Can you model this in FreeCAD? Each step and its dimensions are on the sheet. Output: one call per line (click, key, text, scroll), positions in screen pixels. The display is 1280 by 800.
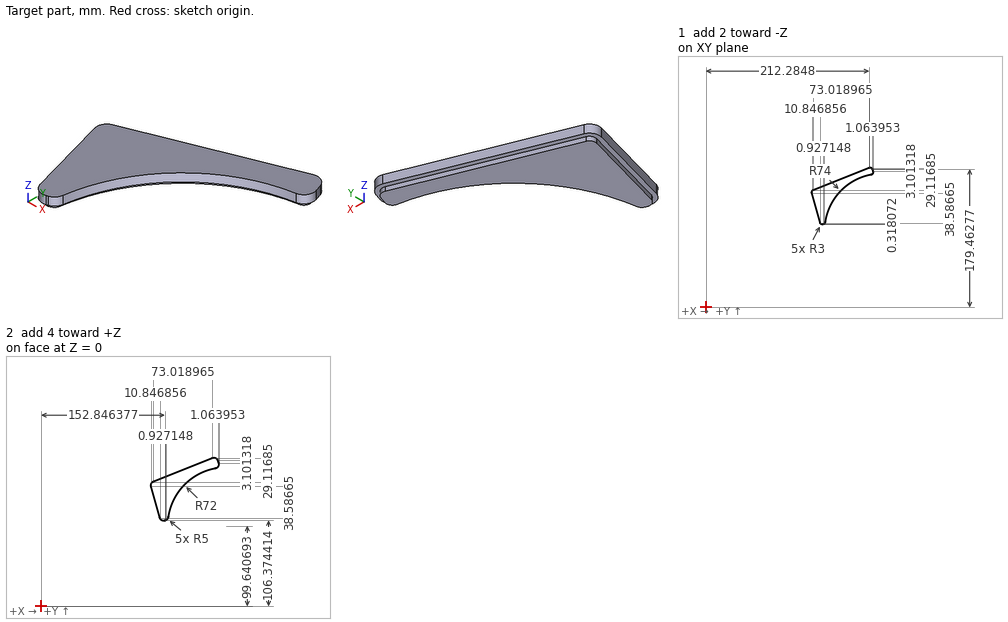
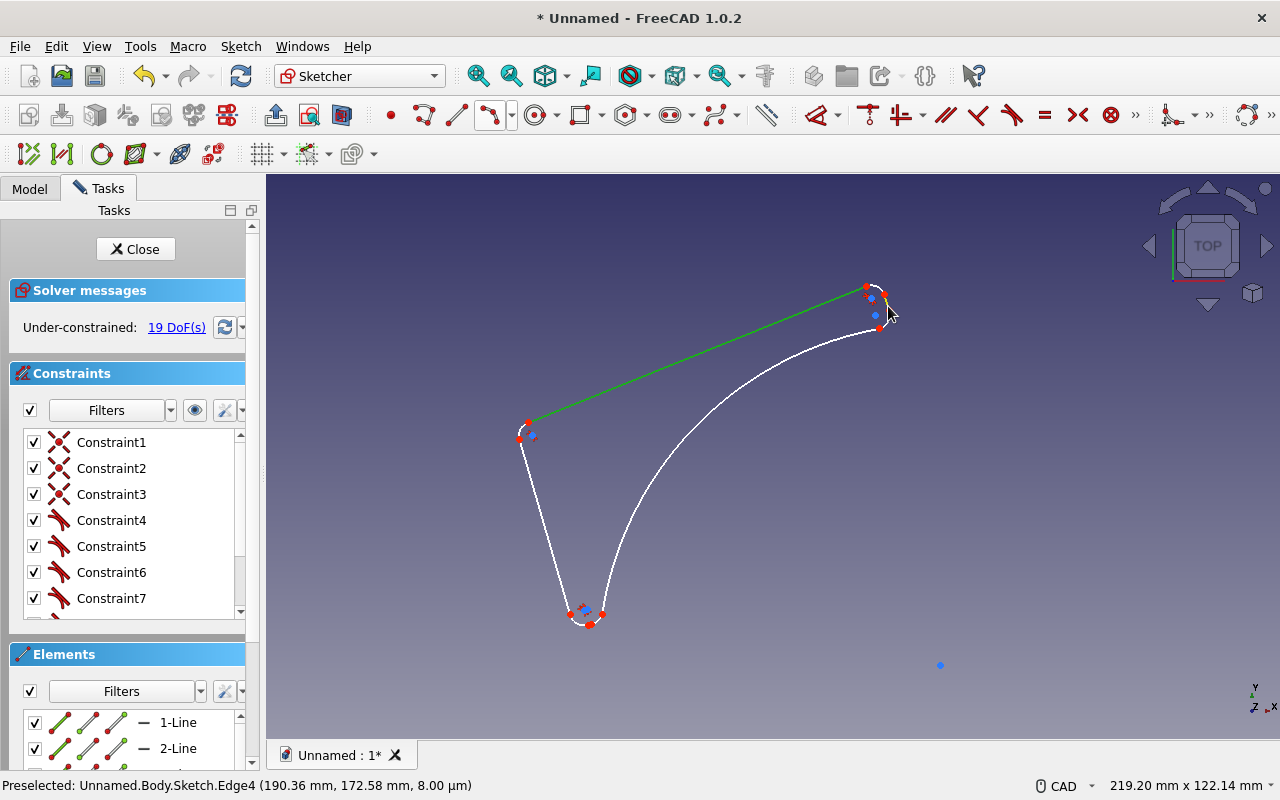
scroll(523, 426, up, 5)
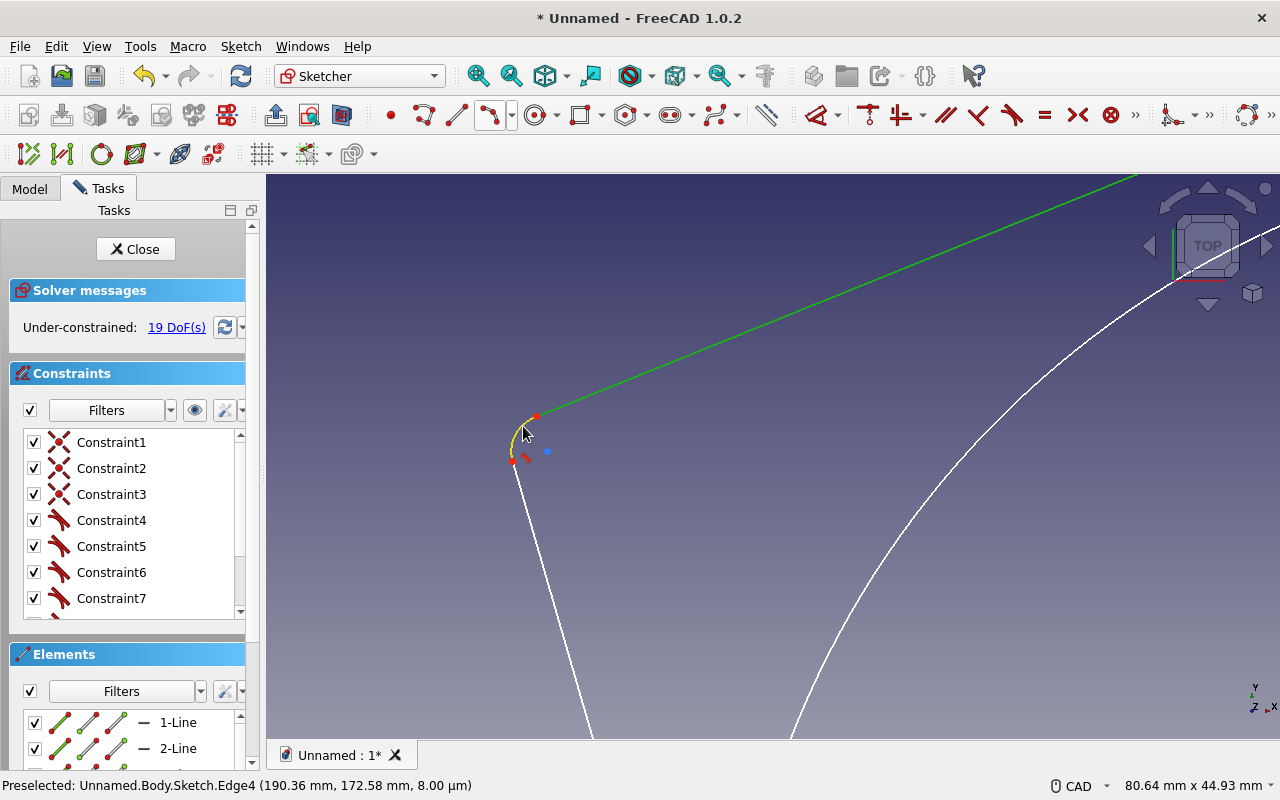
click(522, 425)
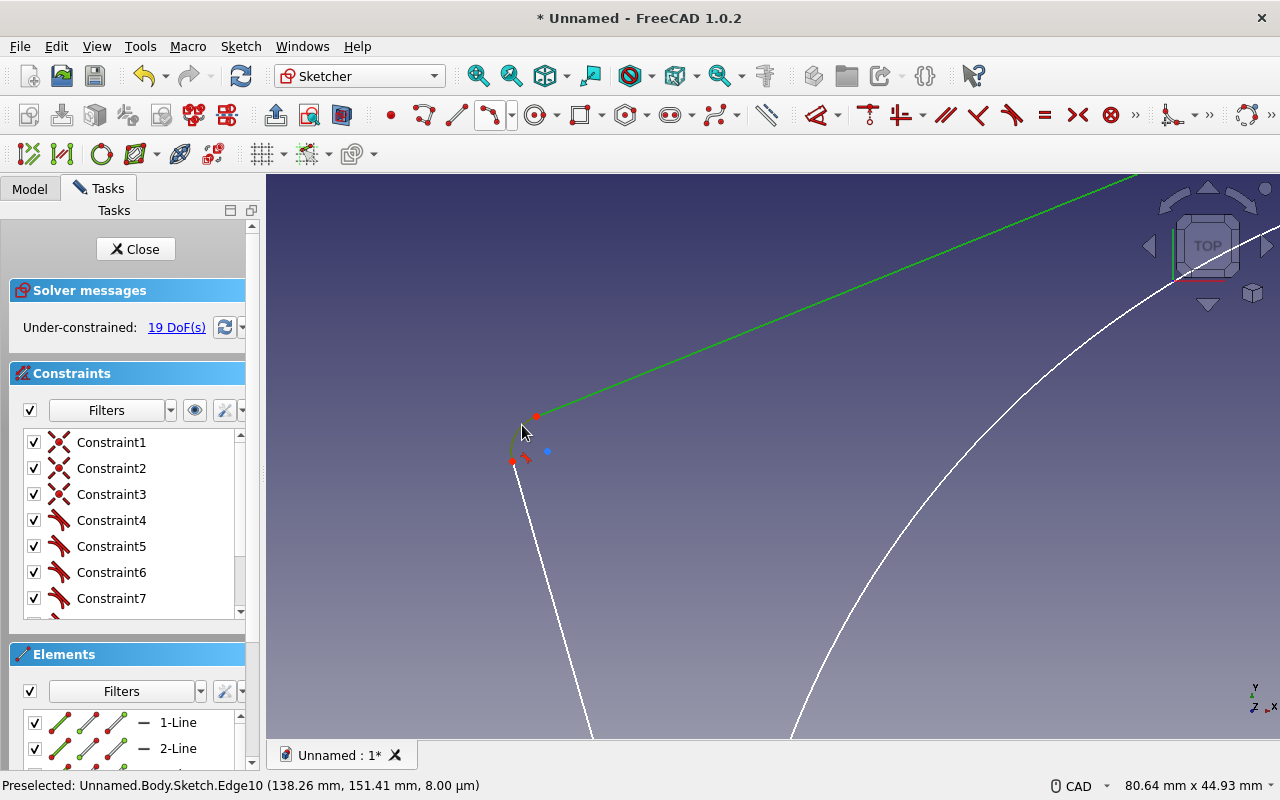
click(1012, 116)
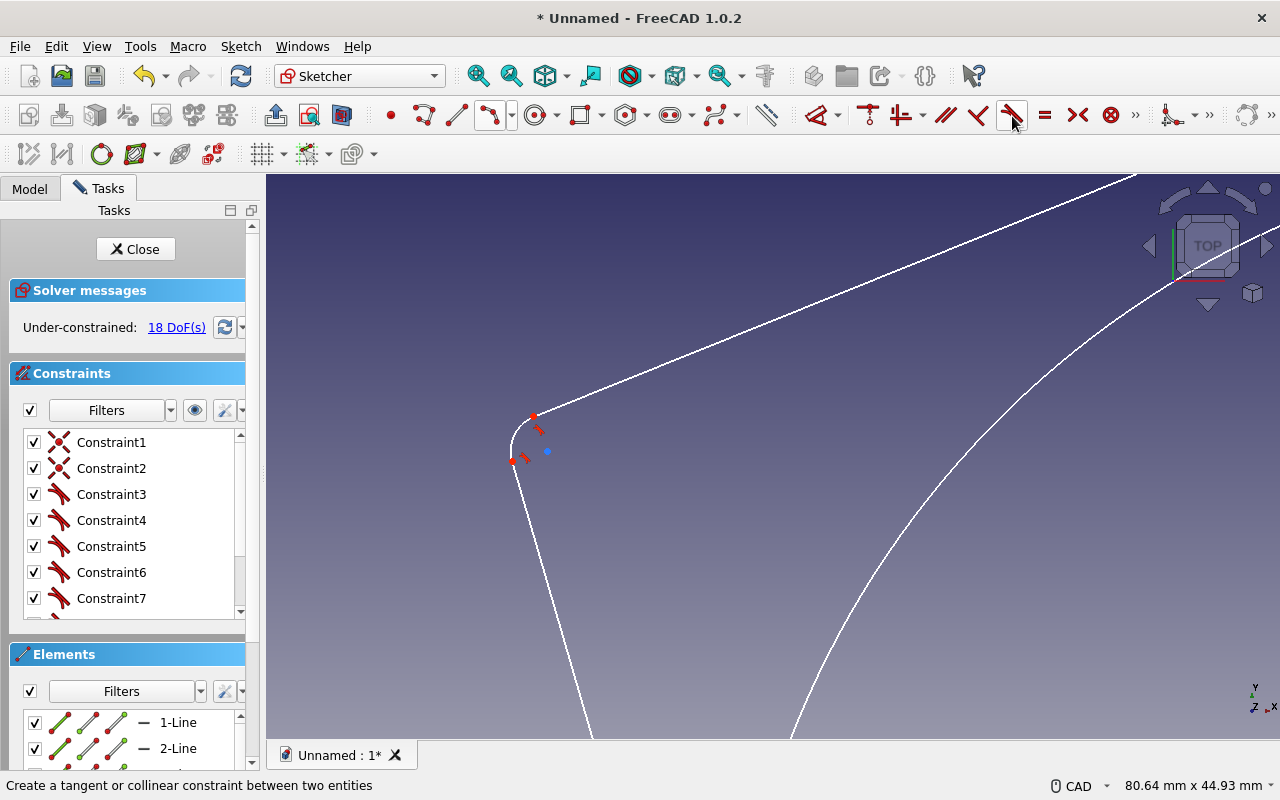
scroll(523, 426, down, 5)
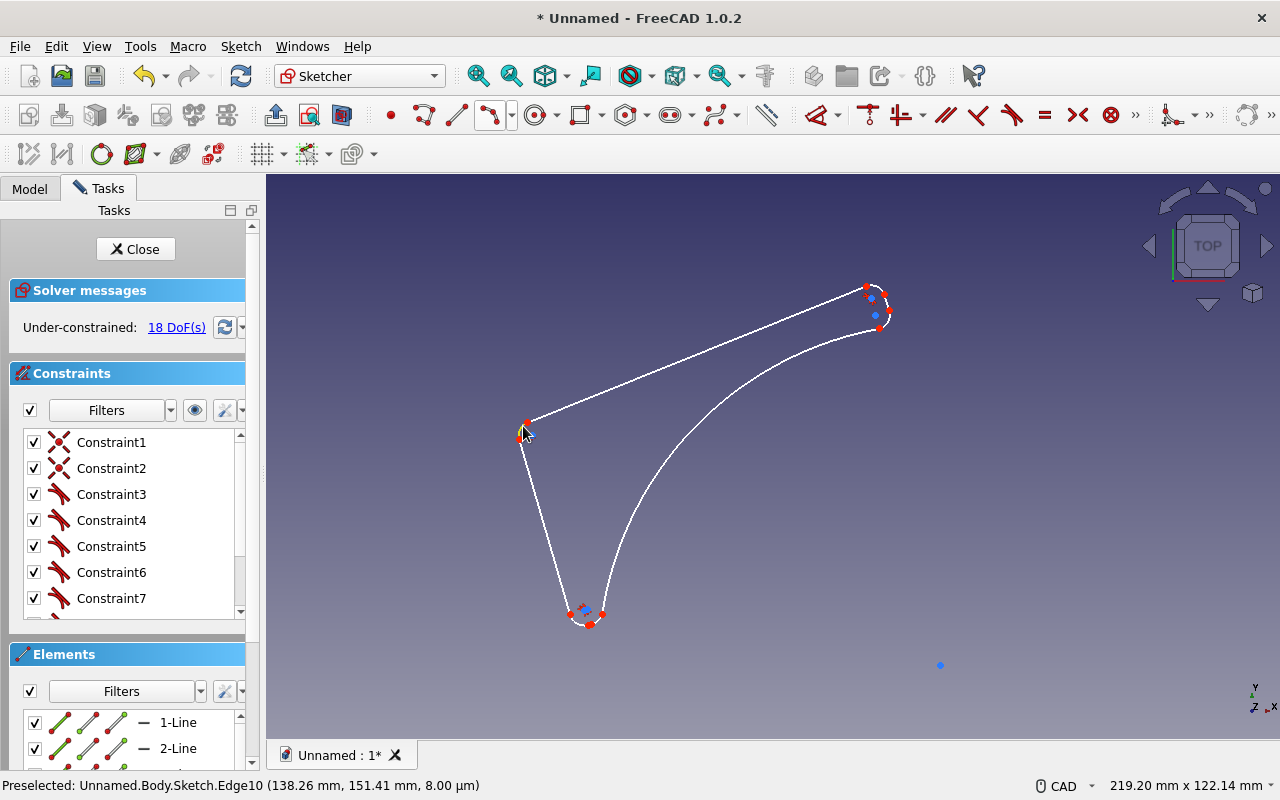
scroll(596, 622, up, 6)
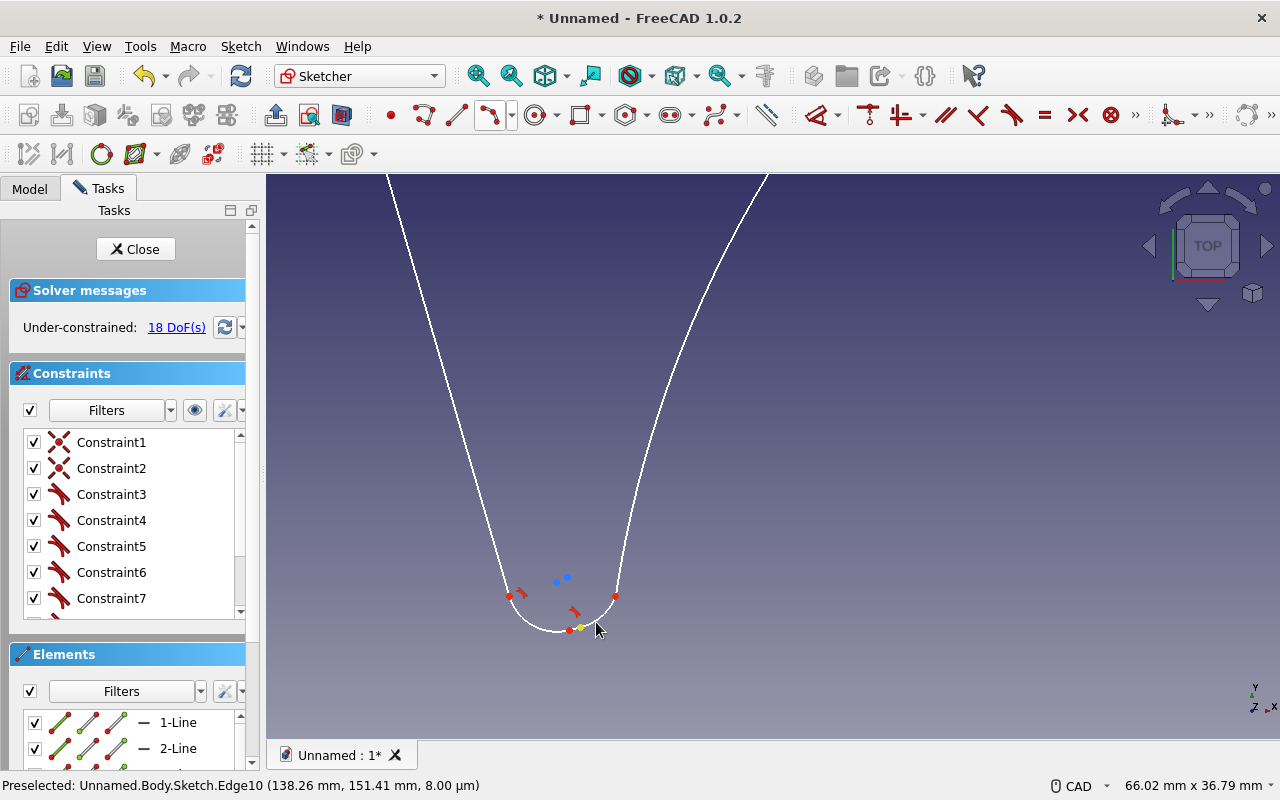
click(594, 622)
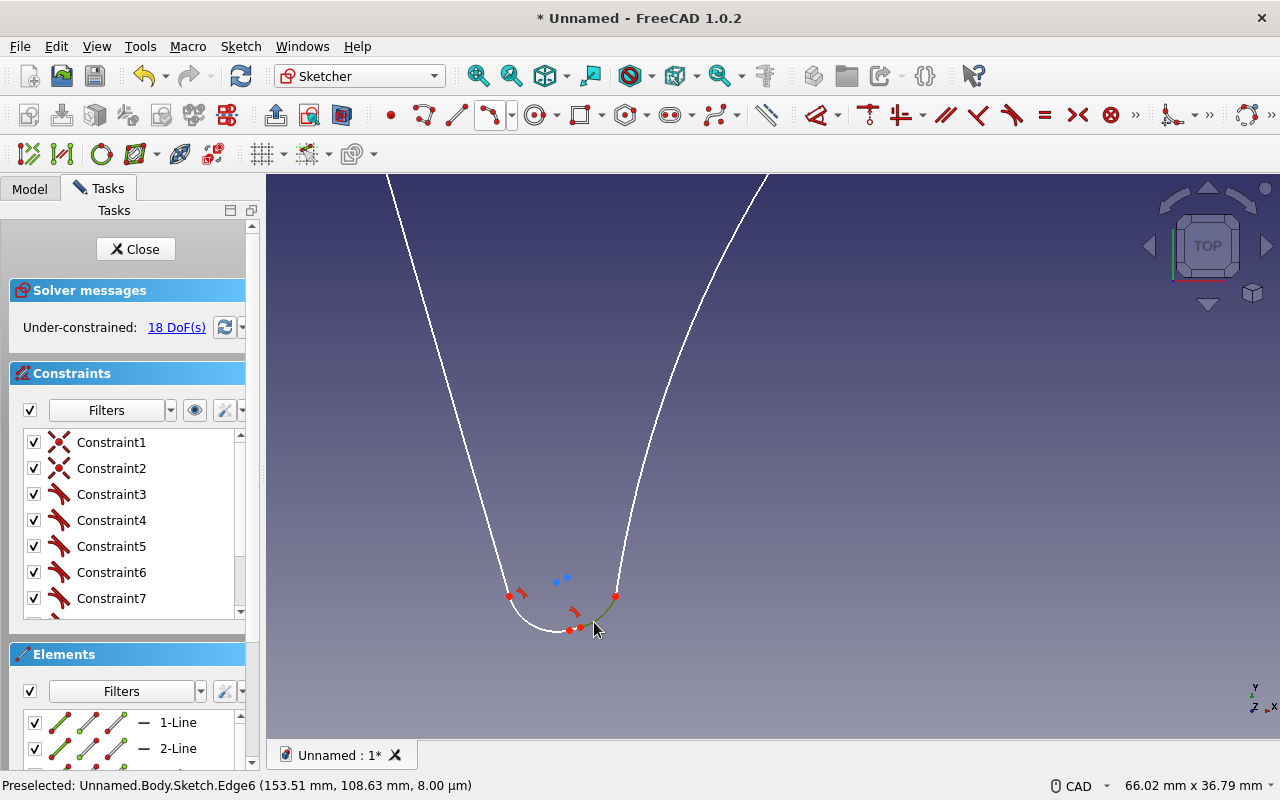
click(691, 325)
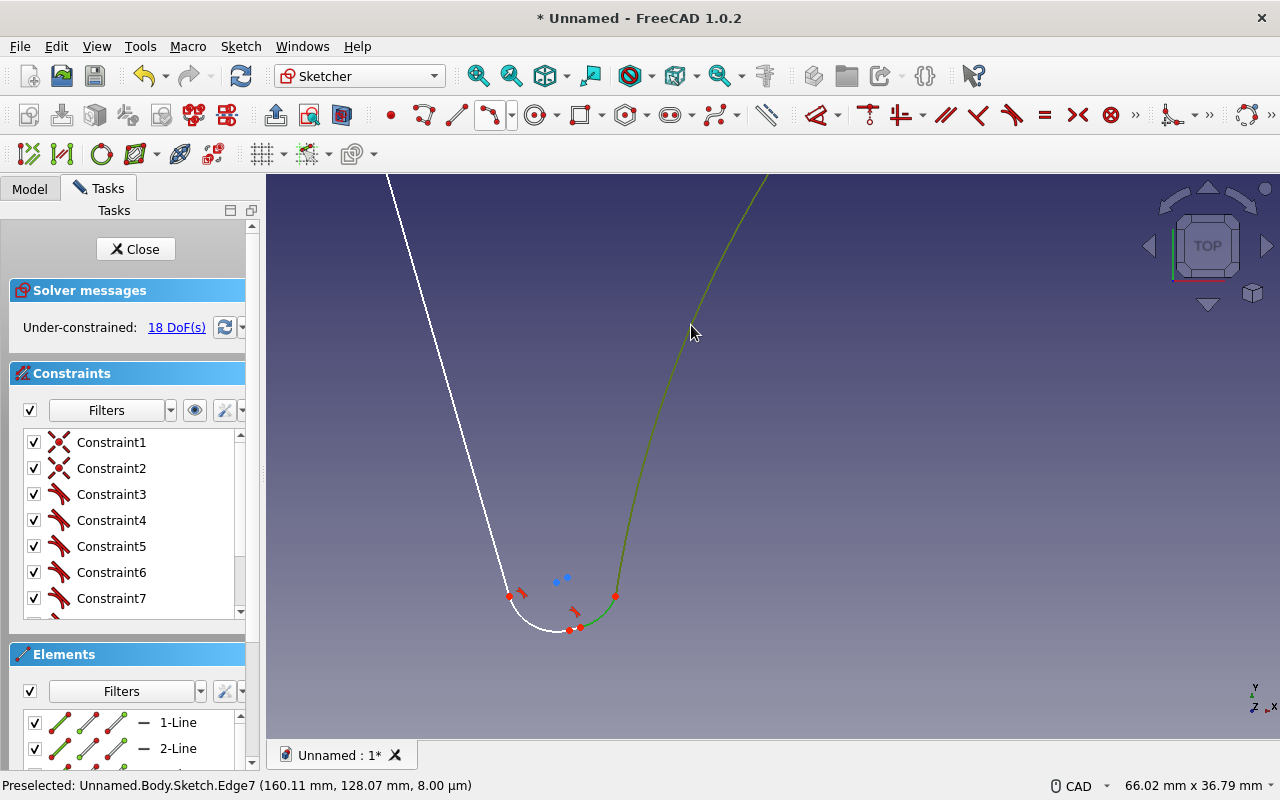
click(1012, 116)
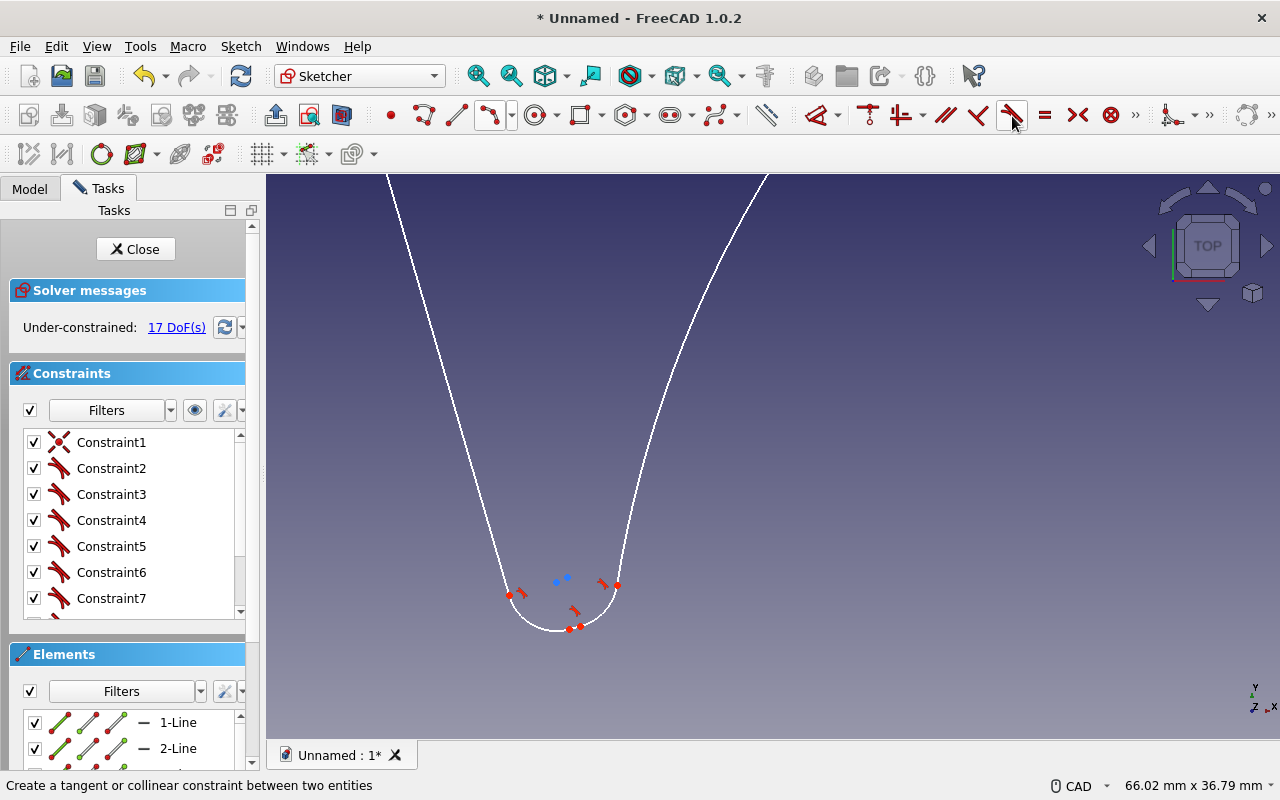
click(694, 317)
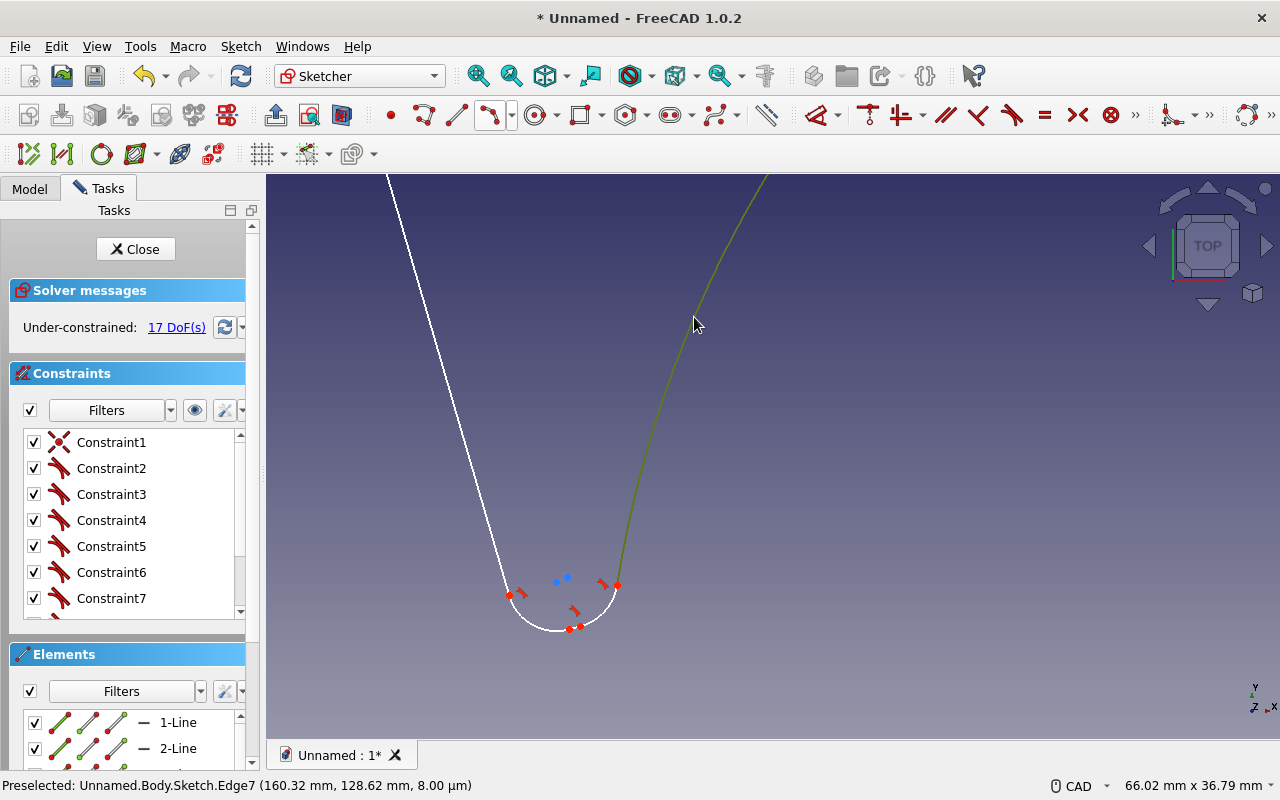
scroll(596, 623, down, 6)